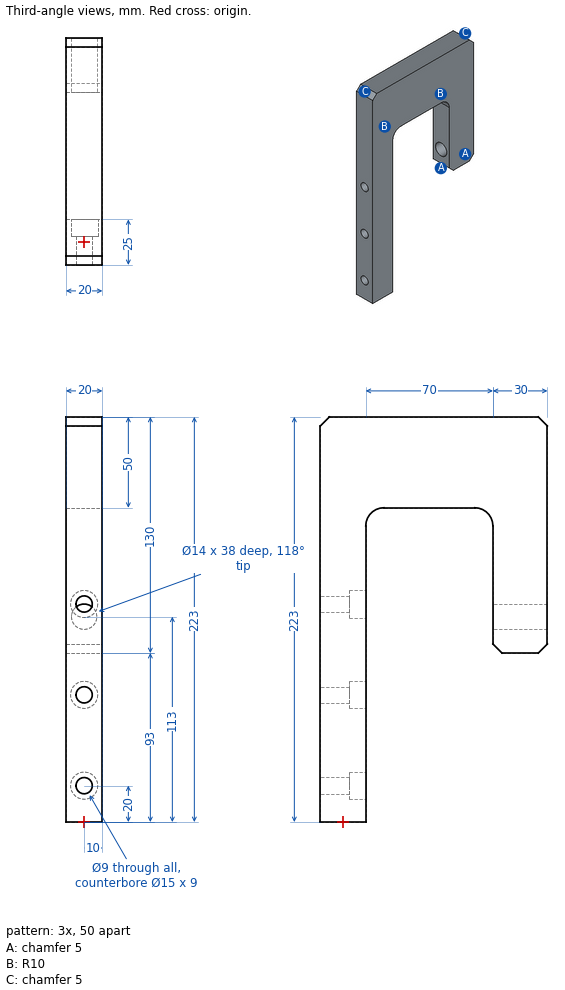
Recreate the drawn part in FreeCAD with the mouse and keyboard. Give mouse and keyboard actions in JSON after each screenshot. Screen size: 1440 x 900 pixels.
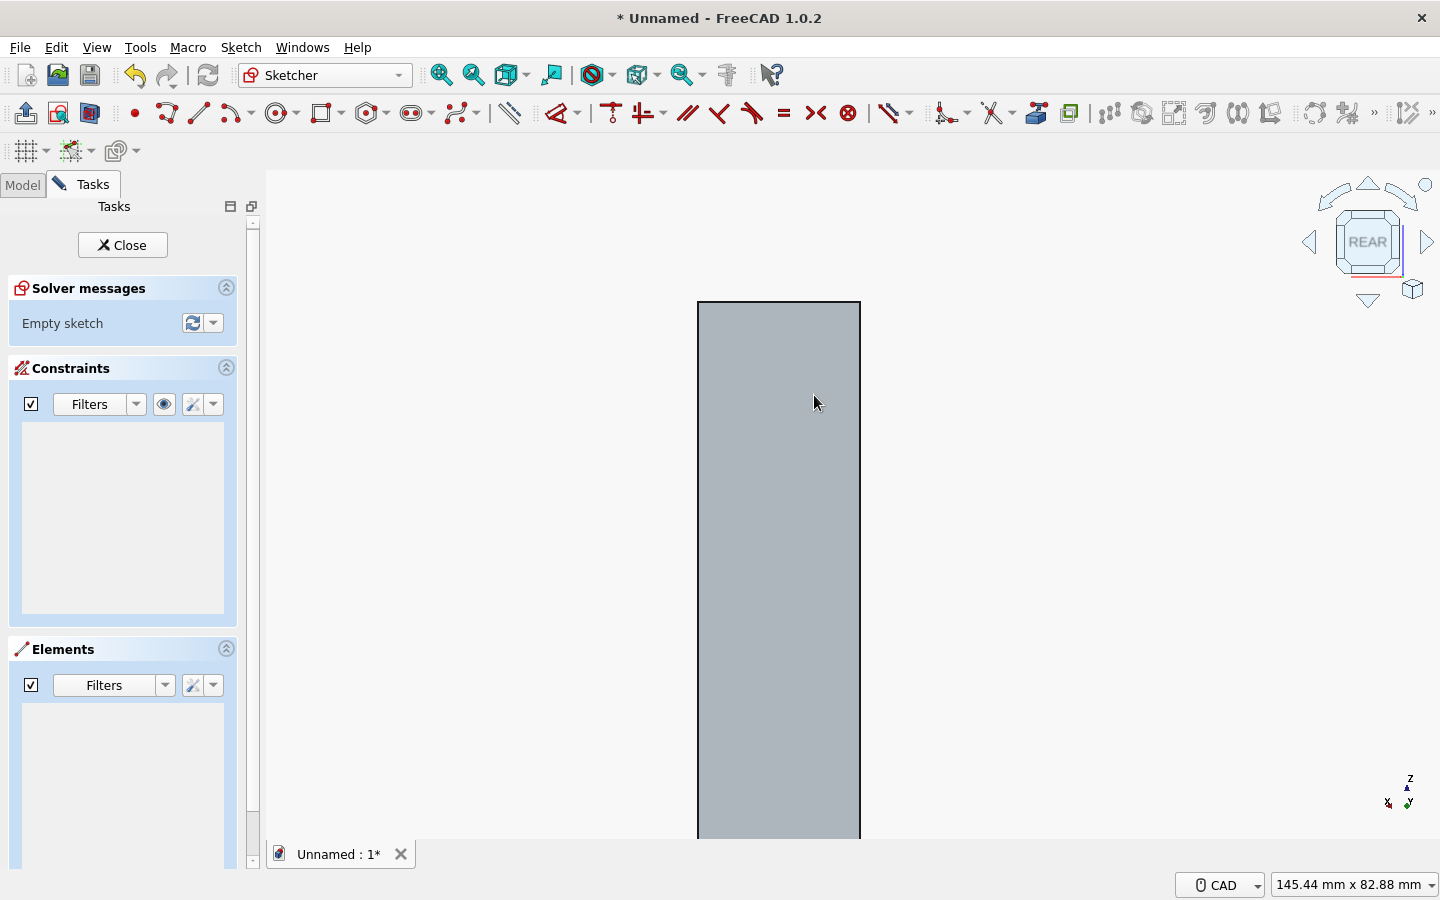
{"action": "left_click", "coordinate": [322, 114]}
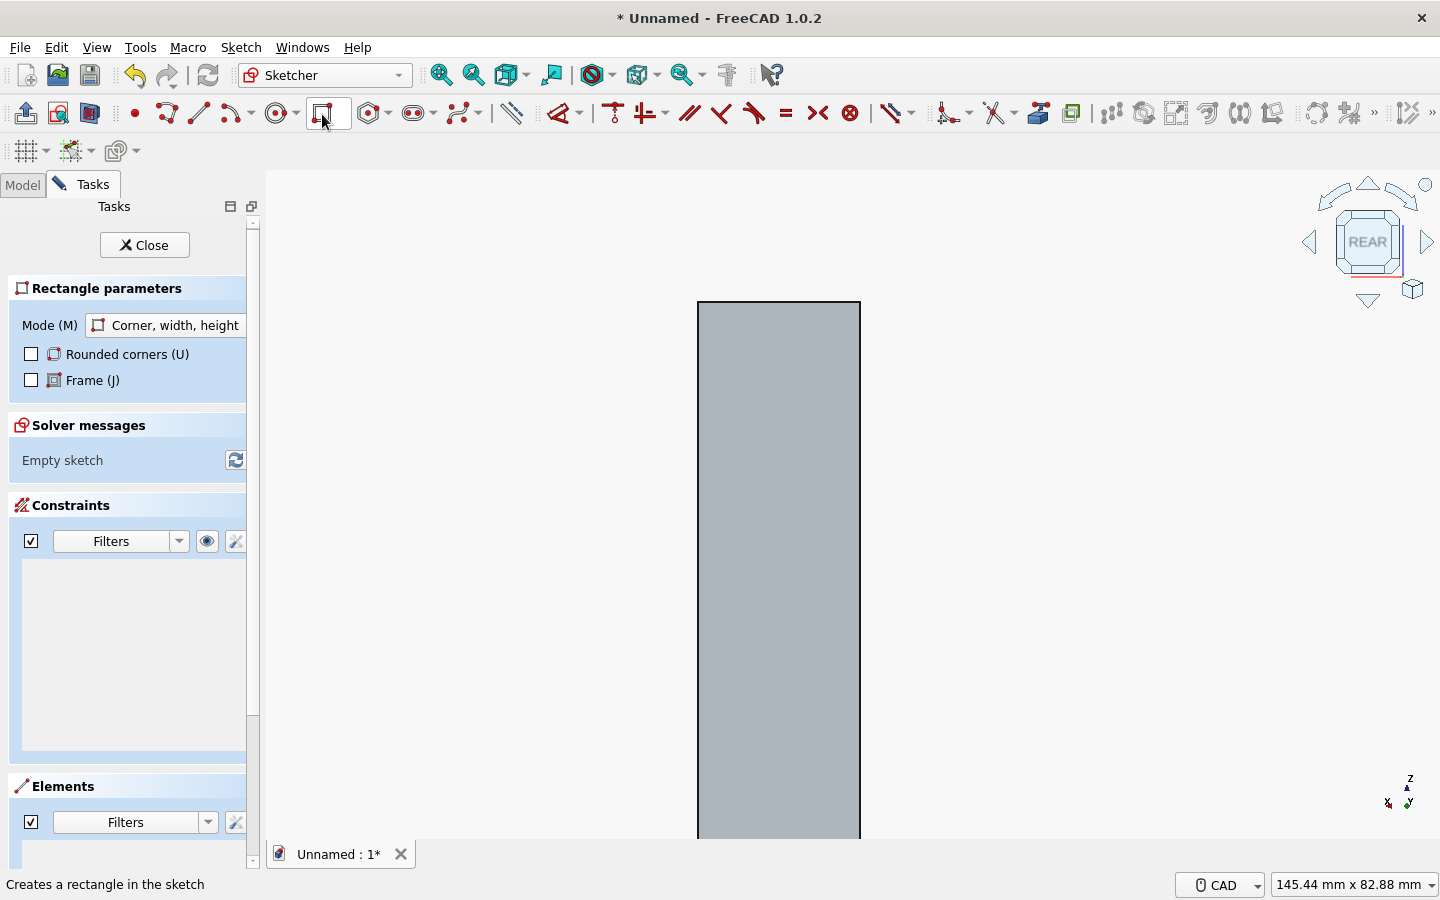
{"action": "left_click", "coordinate": [698, 302]}
{"action": "left_click", "coordinate": [860, 706]}
{"action": "key", "text": "Escape"}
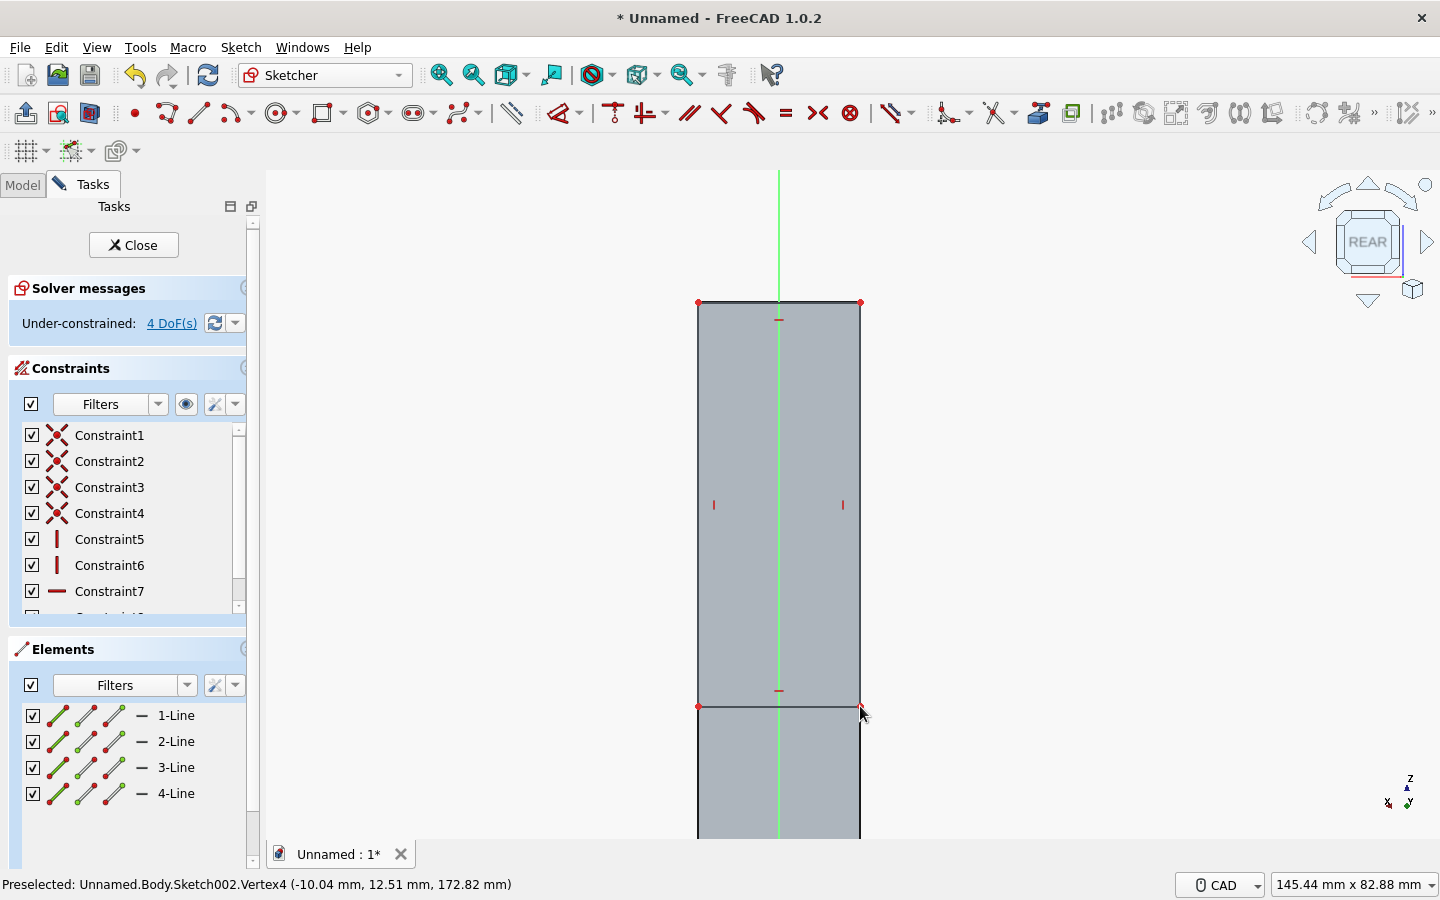
{"action": "left_click", "coordinate": [558, 114]}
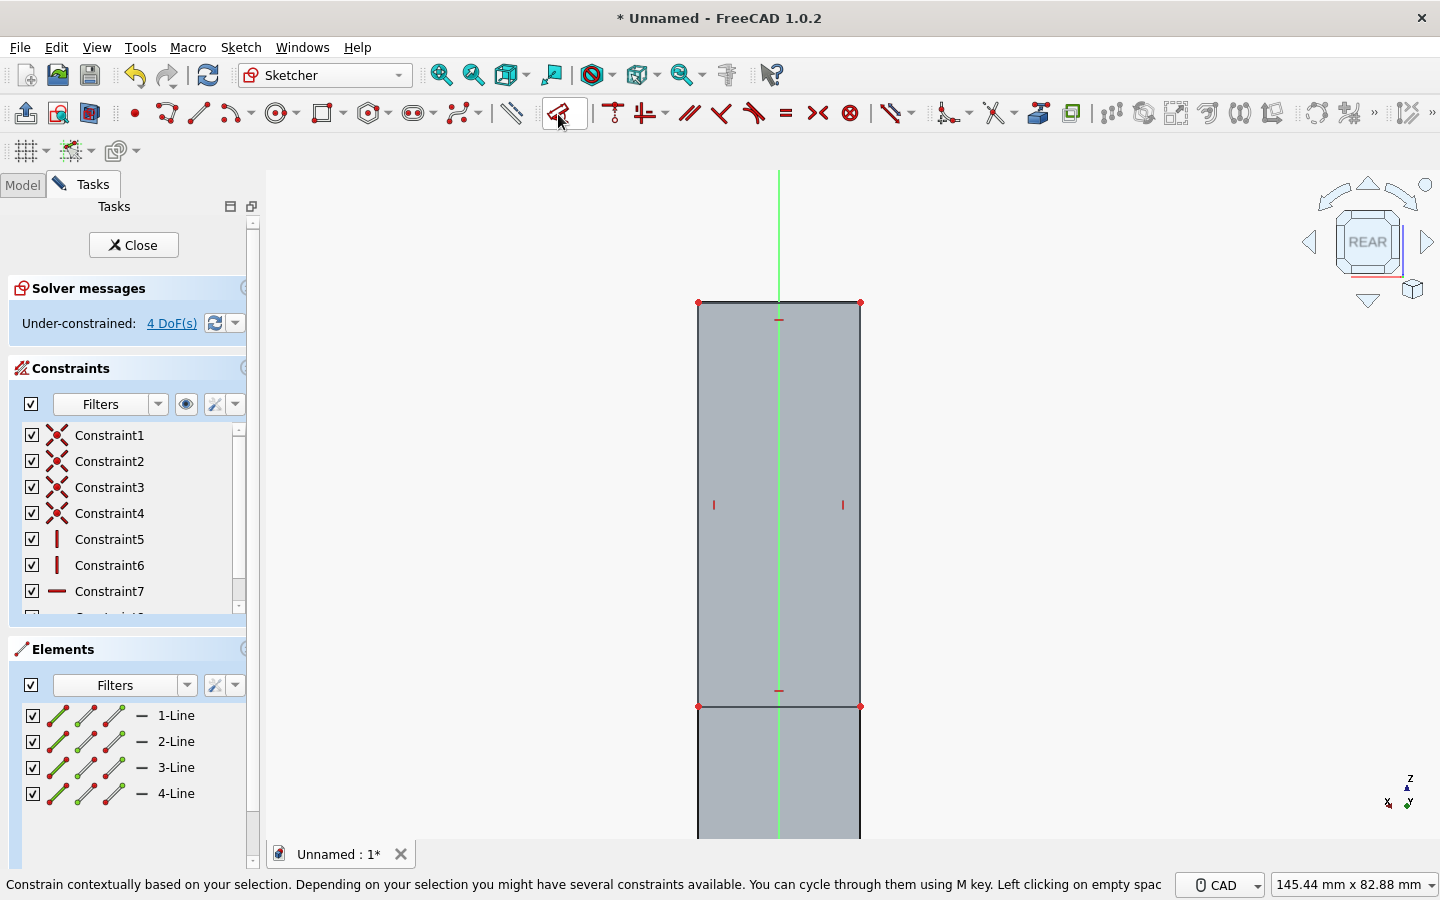
{"action": "left_click", "coordinate": [698, 424]}
{"action": "left_click", "coordinate": [664, 505]}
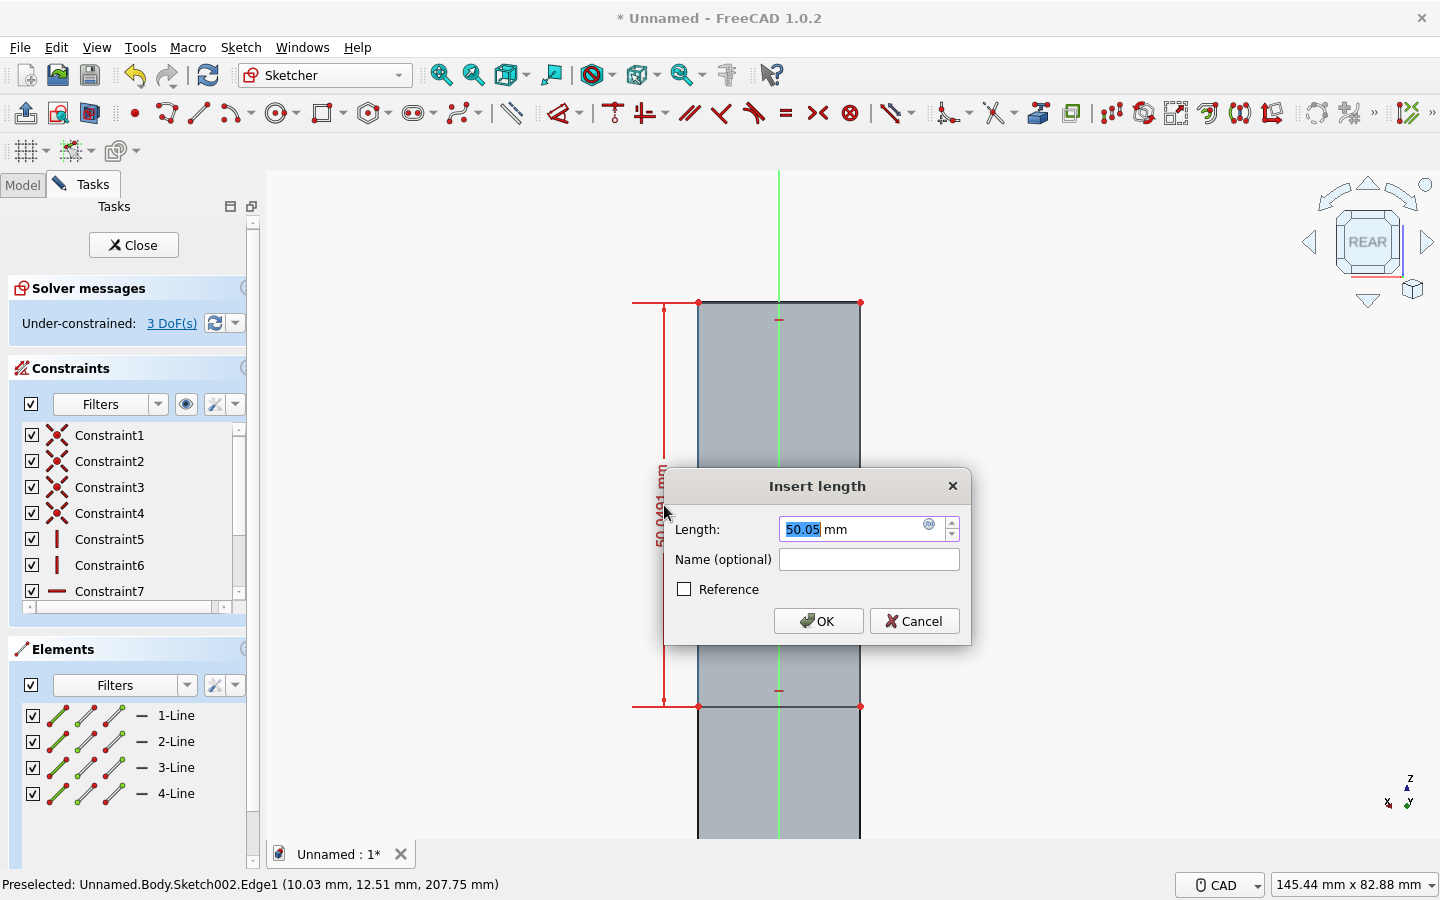
{"action": "type", "text": "50"}
{"action": "key", "text": "Return"}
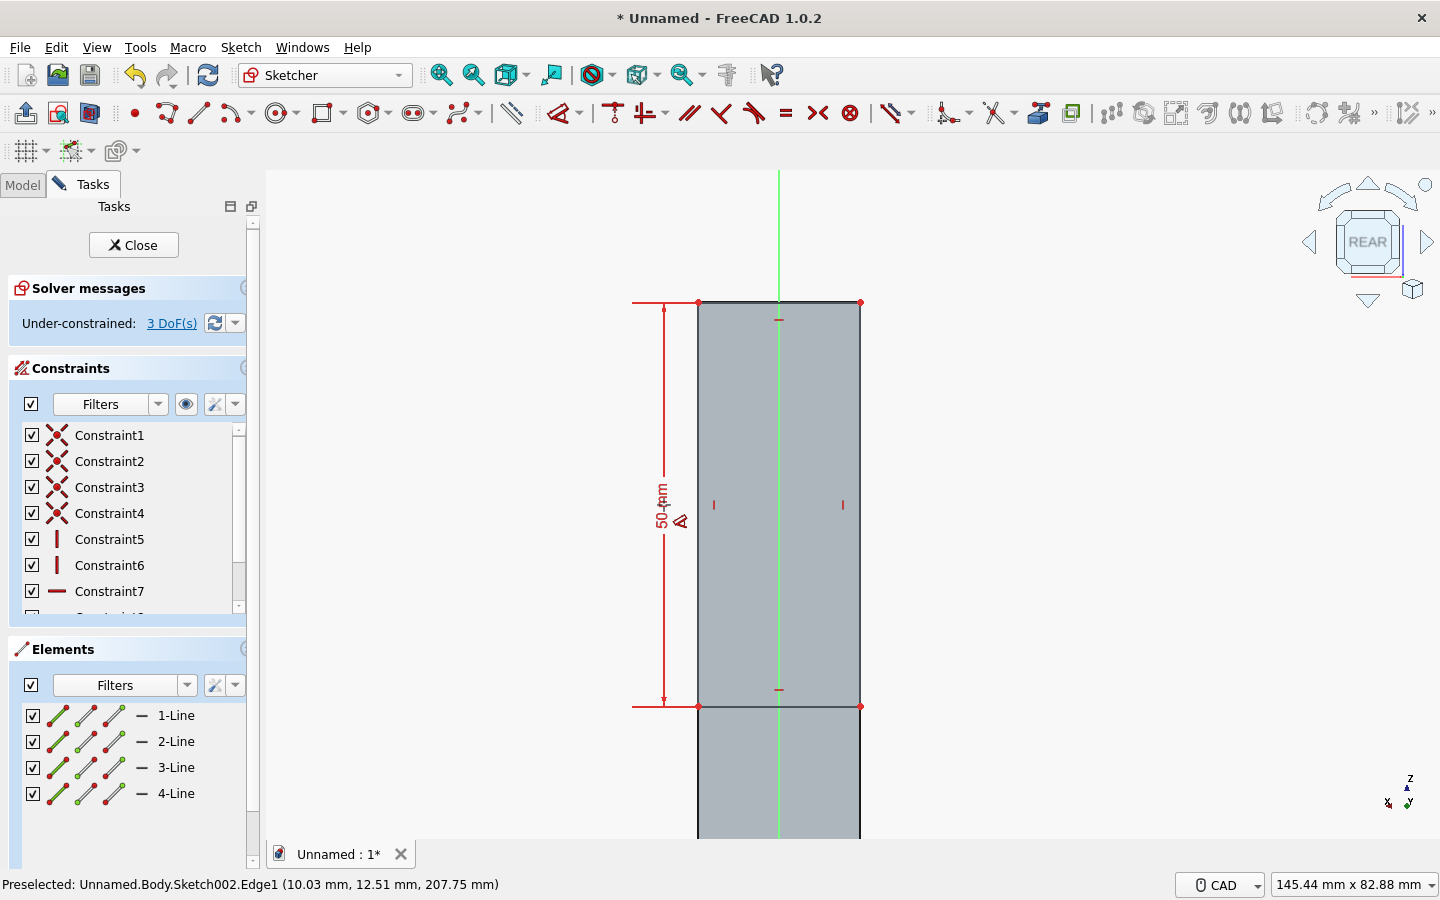
{"action": "left_click", "coordinate": [747, 707]}
{"action": "left_click", "coordinate": [742, 741]}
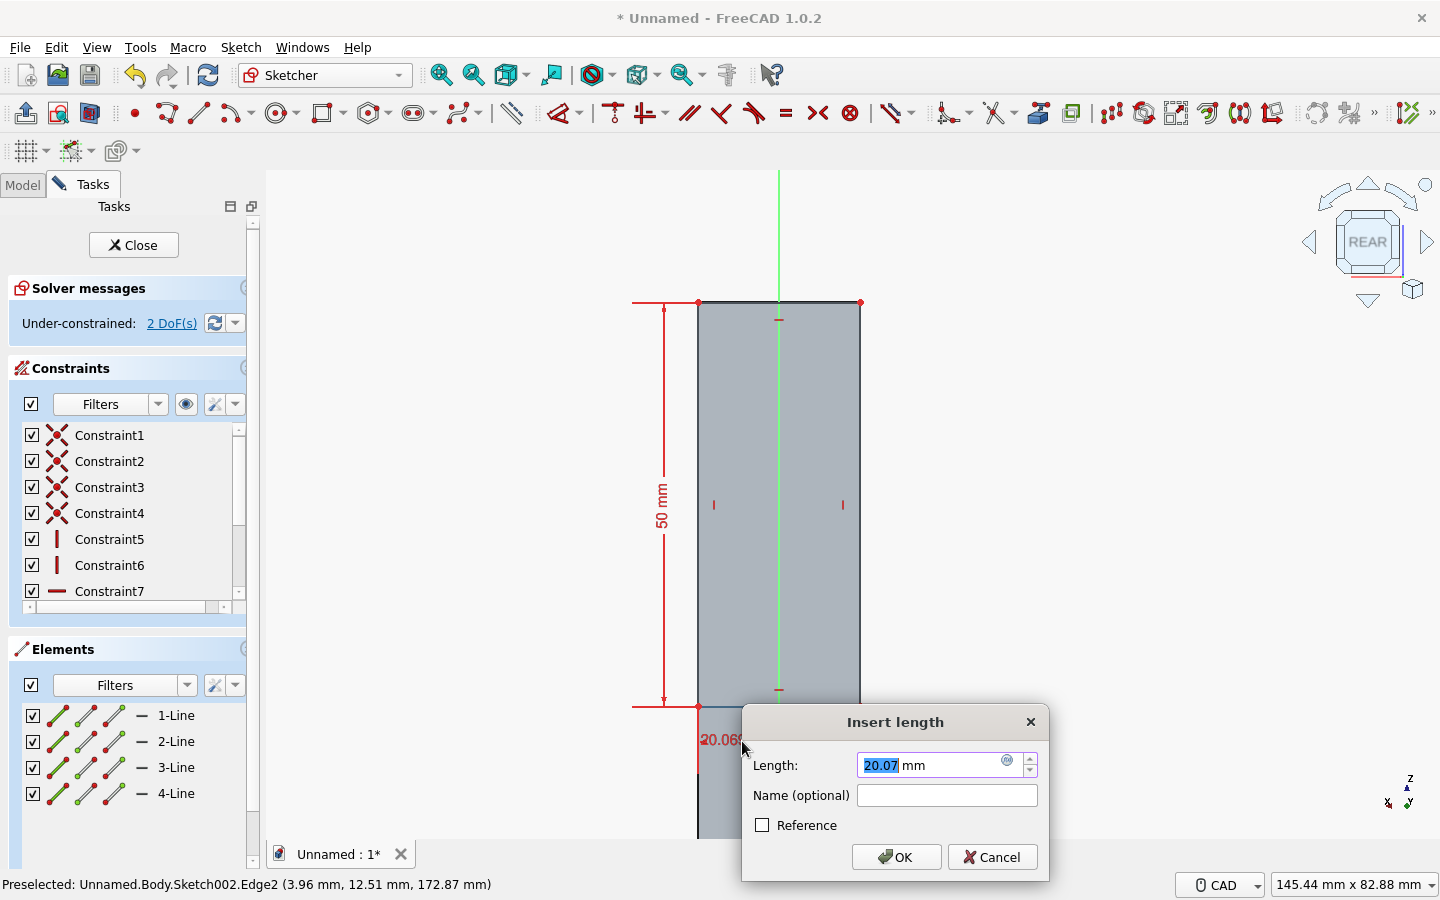
{"action": "type", "text": "20"}
{"action": "key", "text": "Return"}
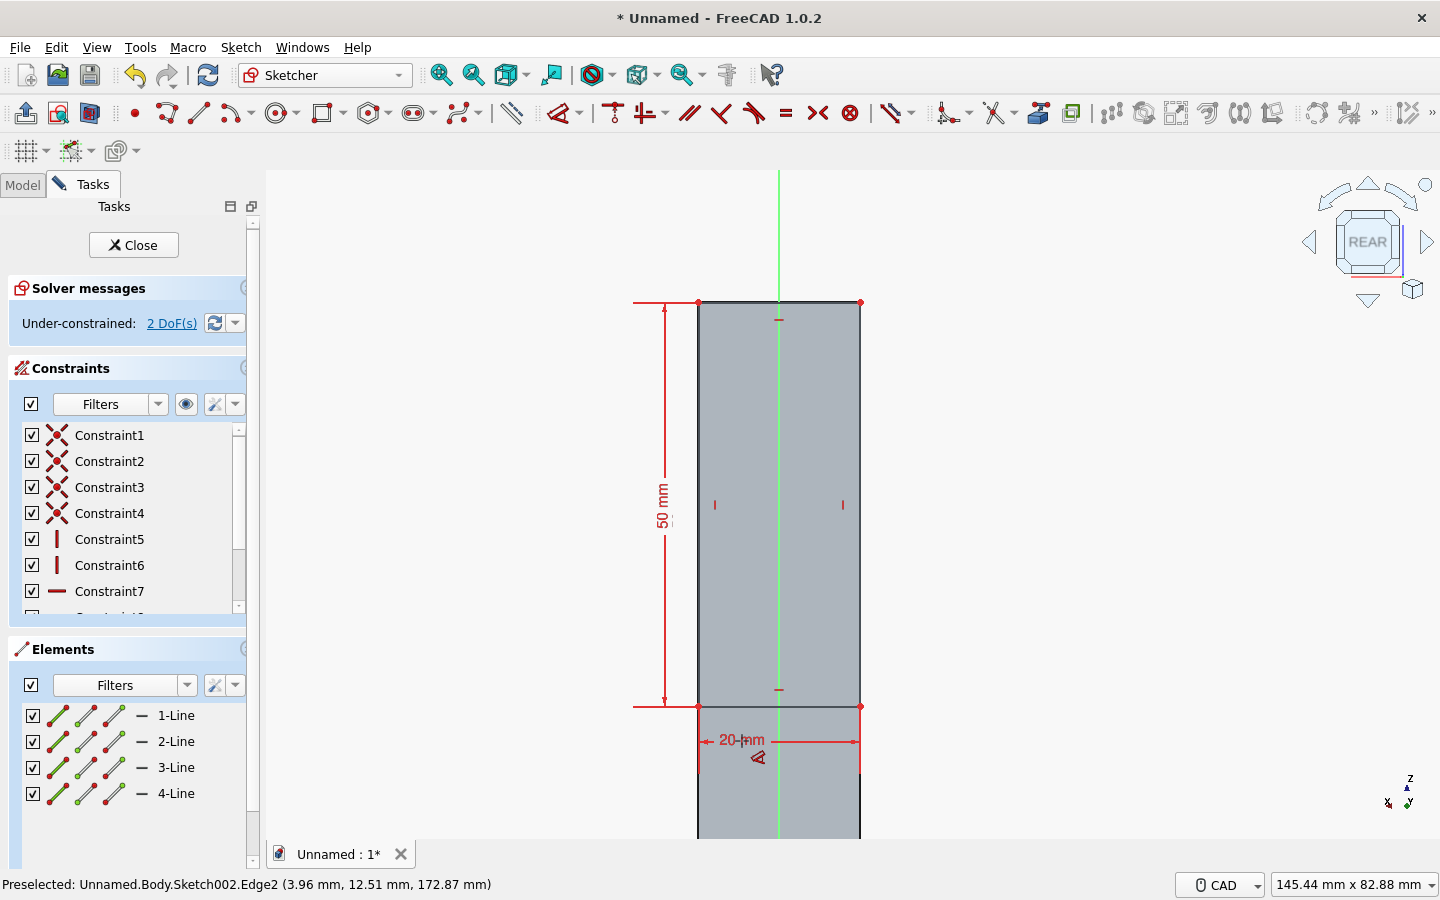
{"action": "left_click", "coordinate": [699, 303]}
{"action": "left_click", "coordinate": [739, 269]}